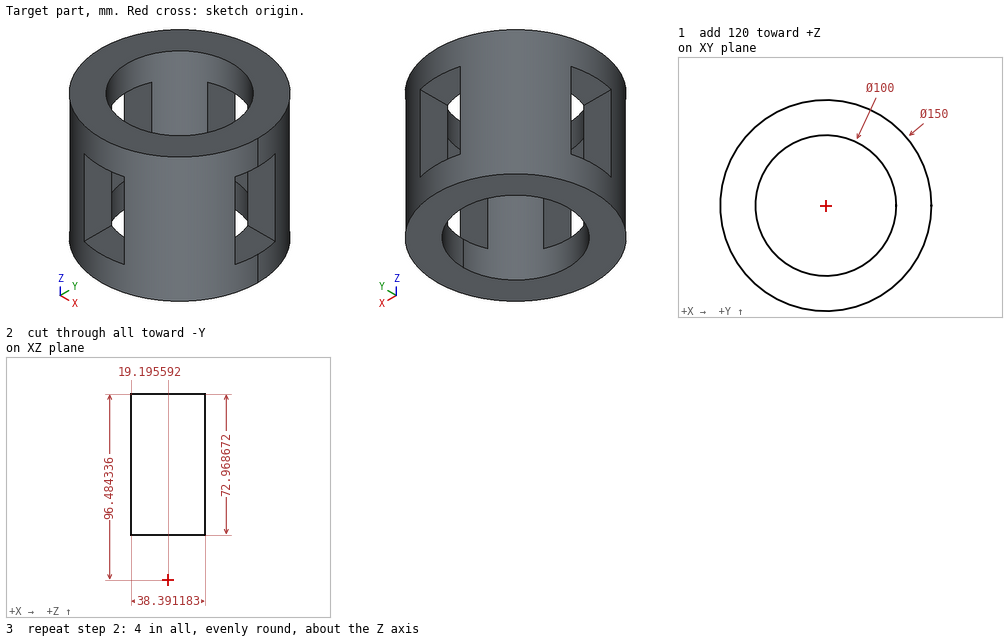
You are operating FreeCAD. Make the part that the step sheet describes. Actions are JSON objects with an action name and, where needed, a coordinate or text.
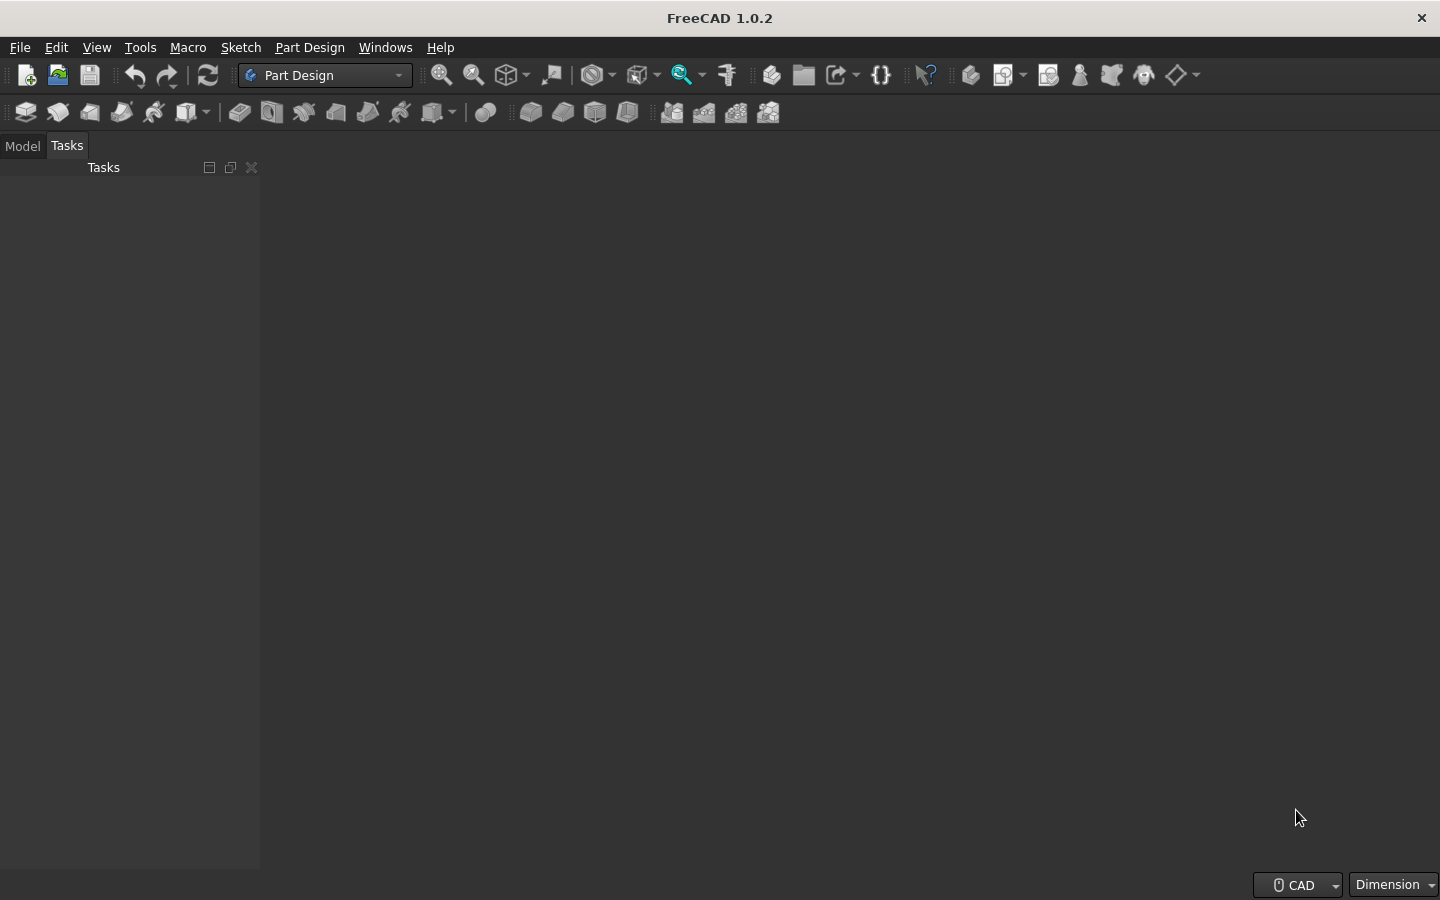
{"action": "left_click", "coordinate": [26, 76]}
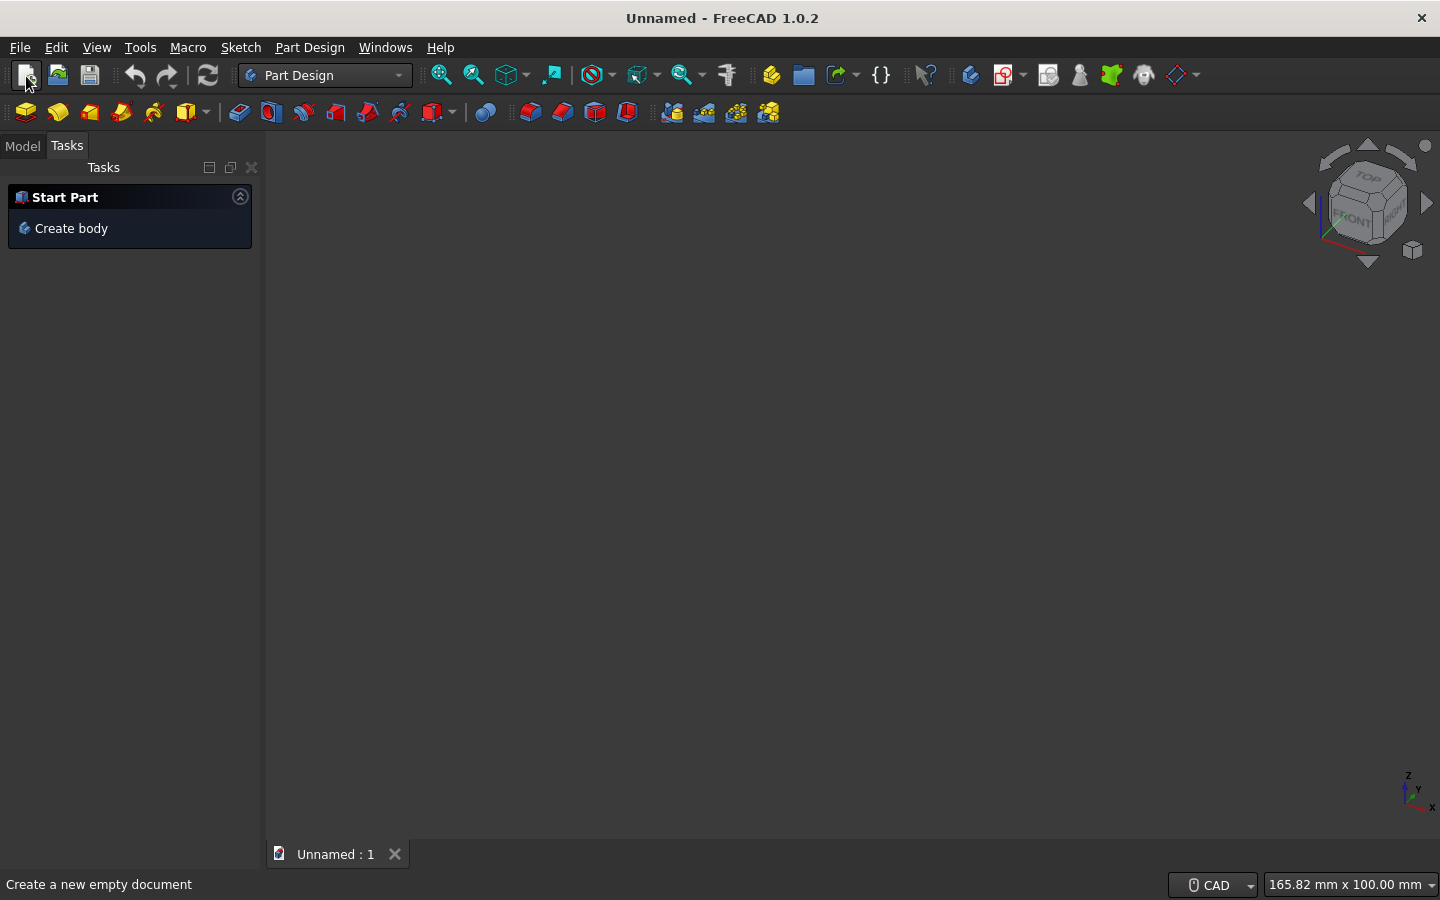
{"action": "left_click", "coordinate": [1004, 76]}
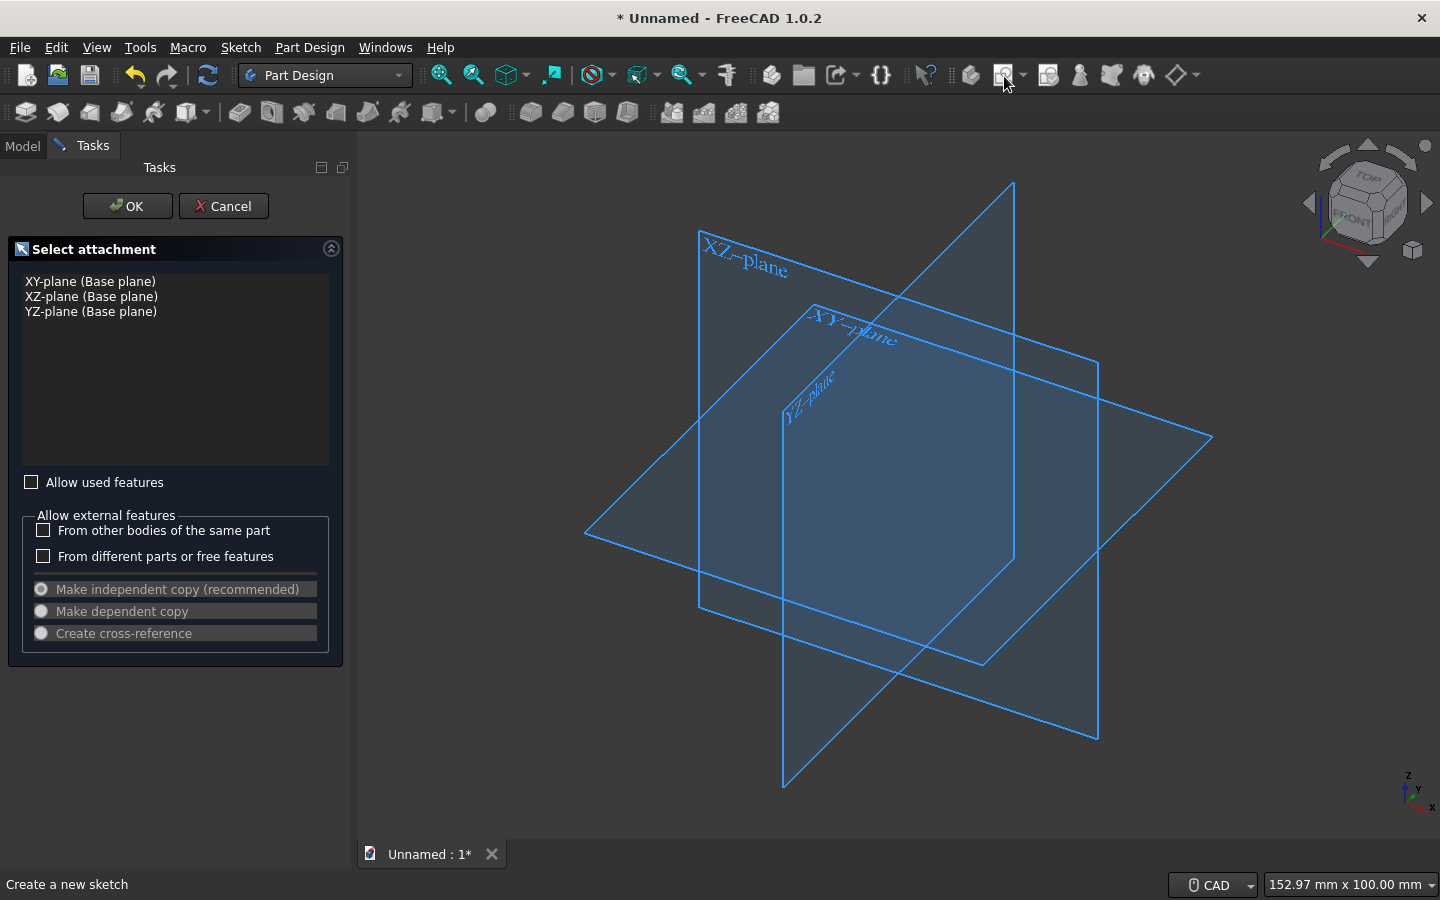
{"action": "left_click", "coordinate": [82, 282]}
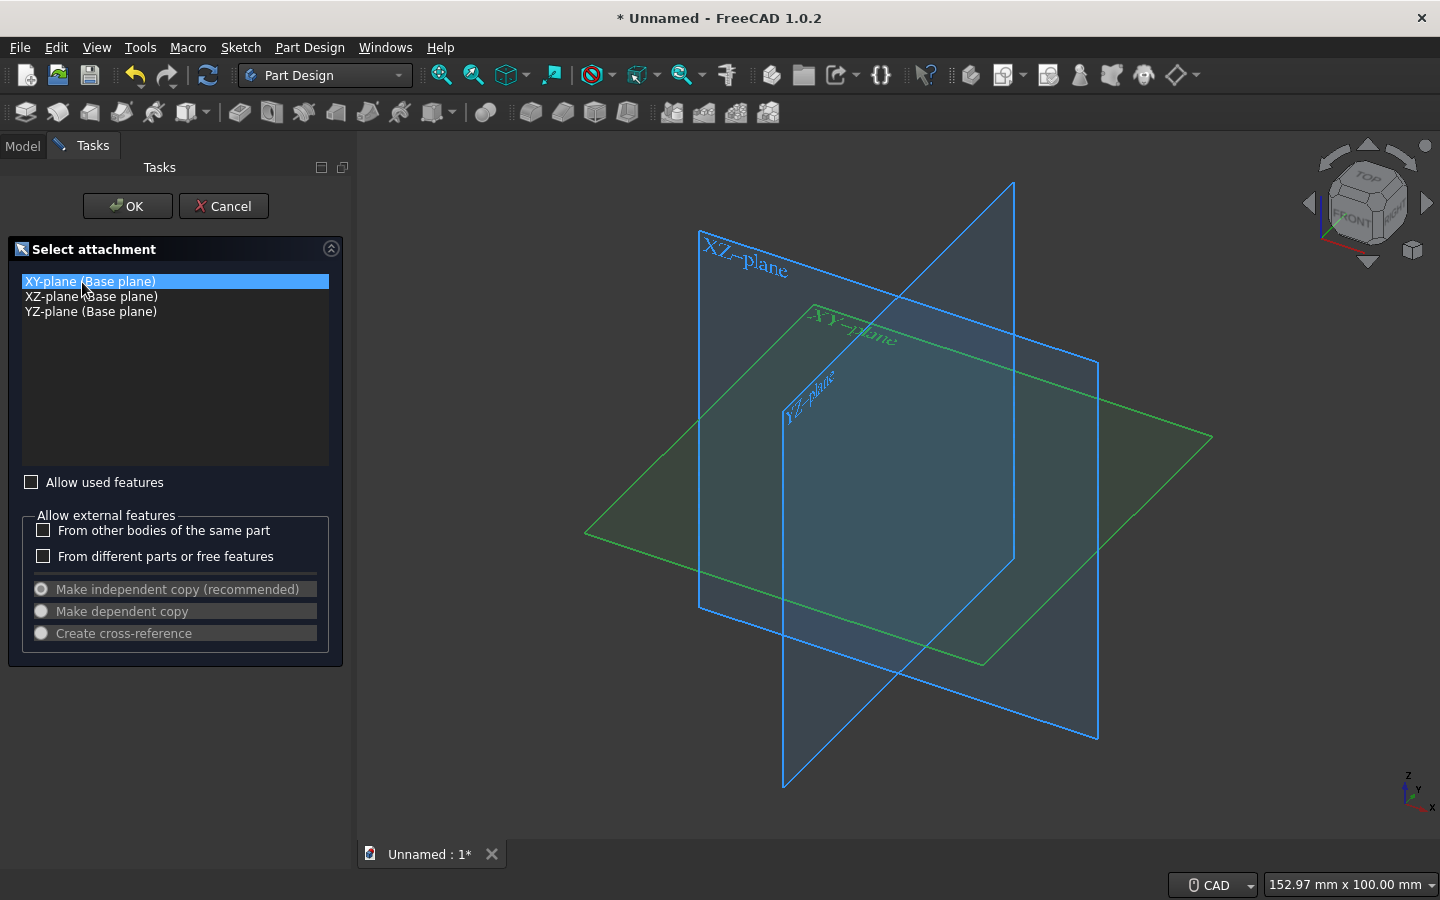
{"action": "left_click", "coordinate": [128, 206]}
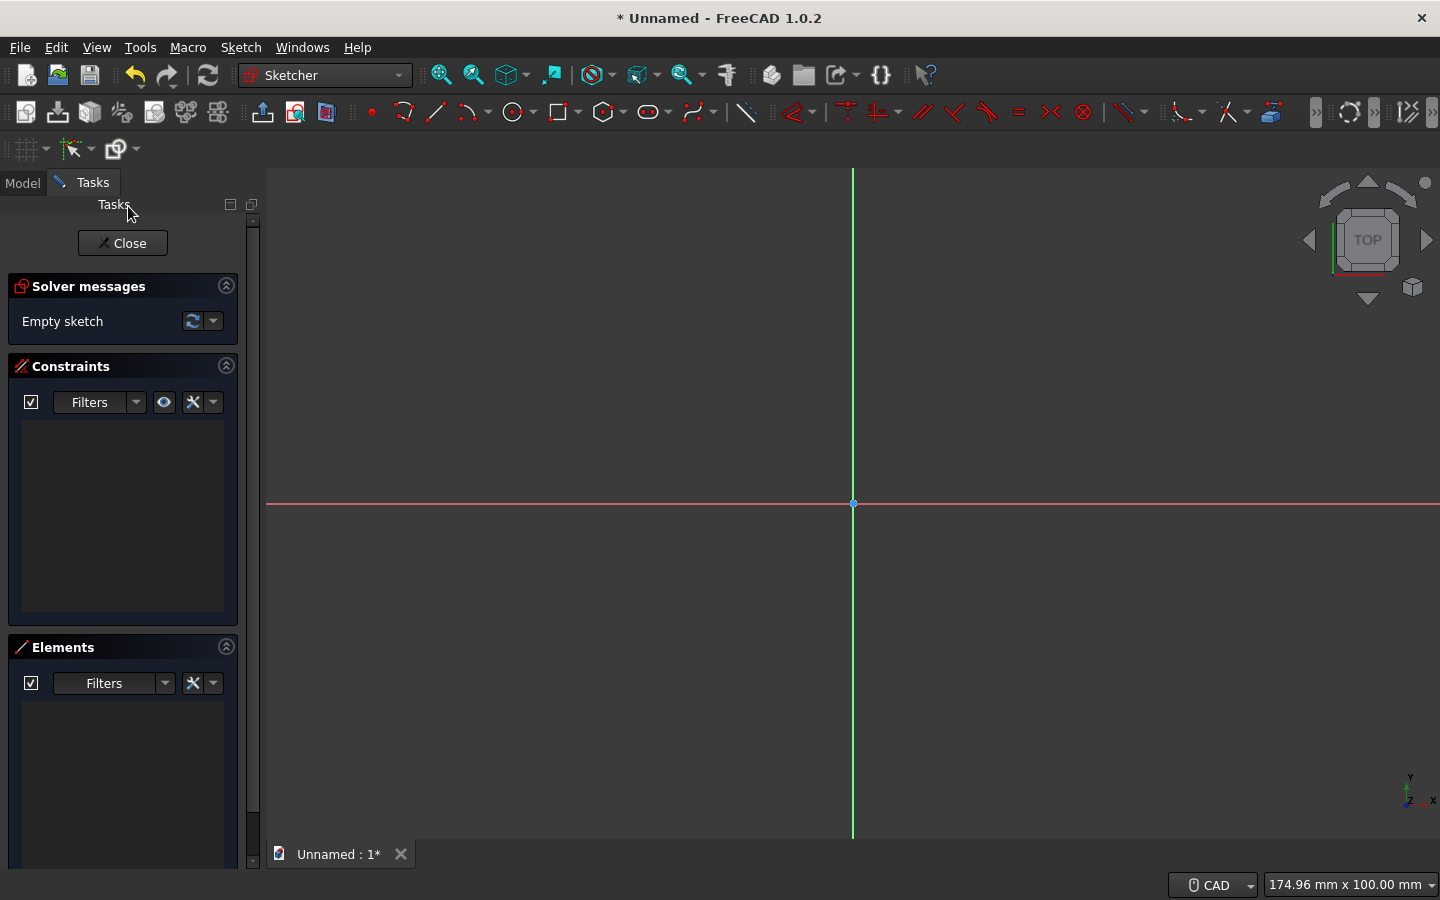
{"action": "scroll", "coordinate": [729, 503], "scroll_direction": "down", "scroll_amount": 4}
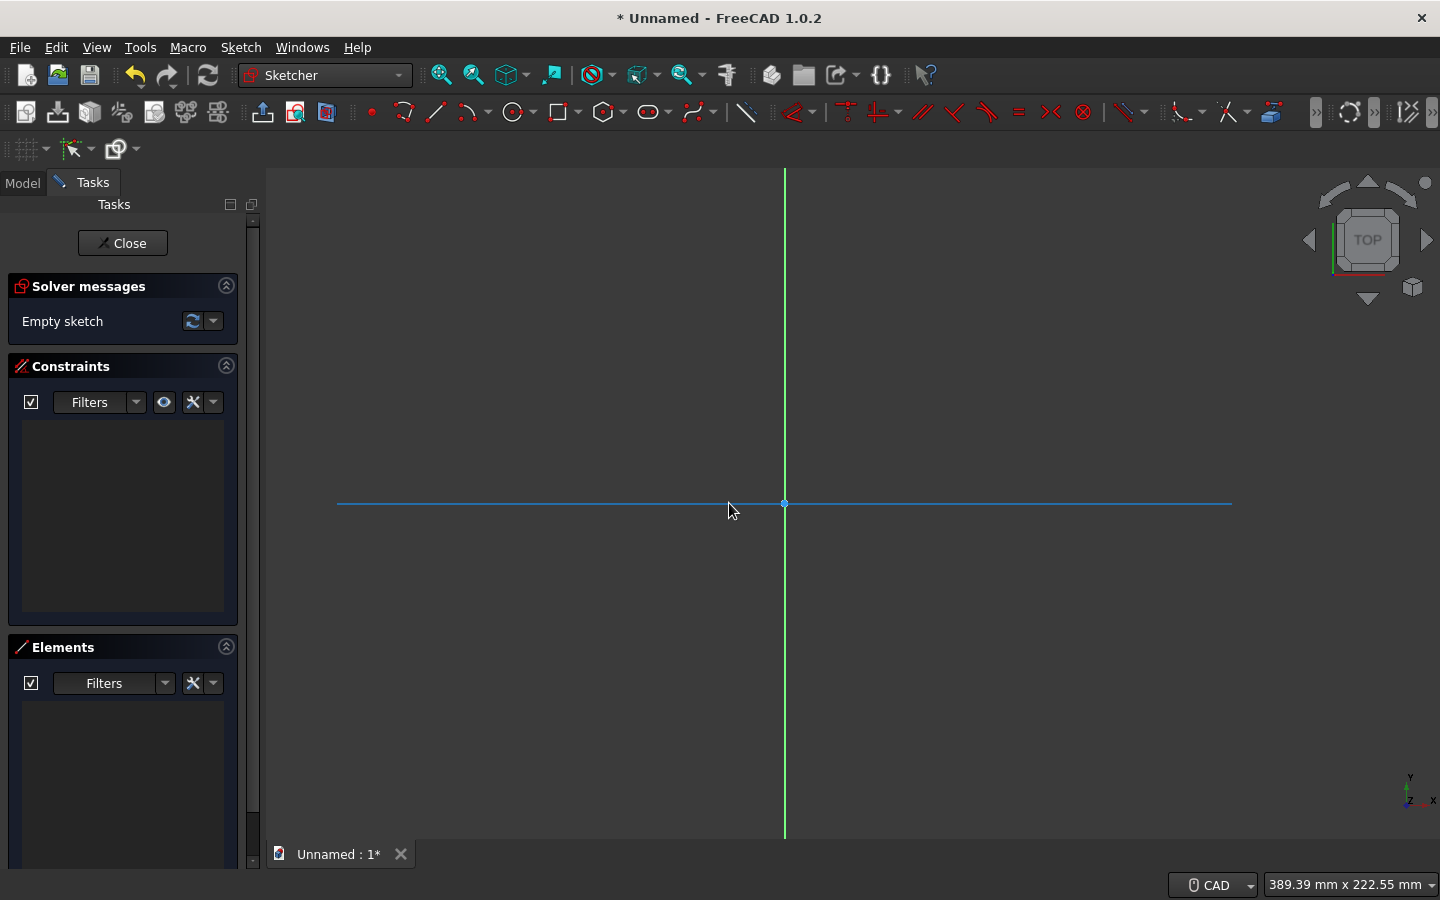
{"action": "left_click", "coordinate": [514, 112]}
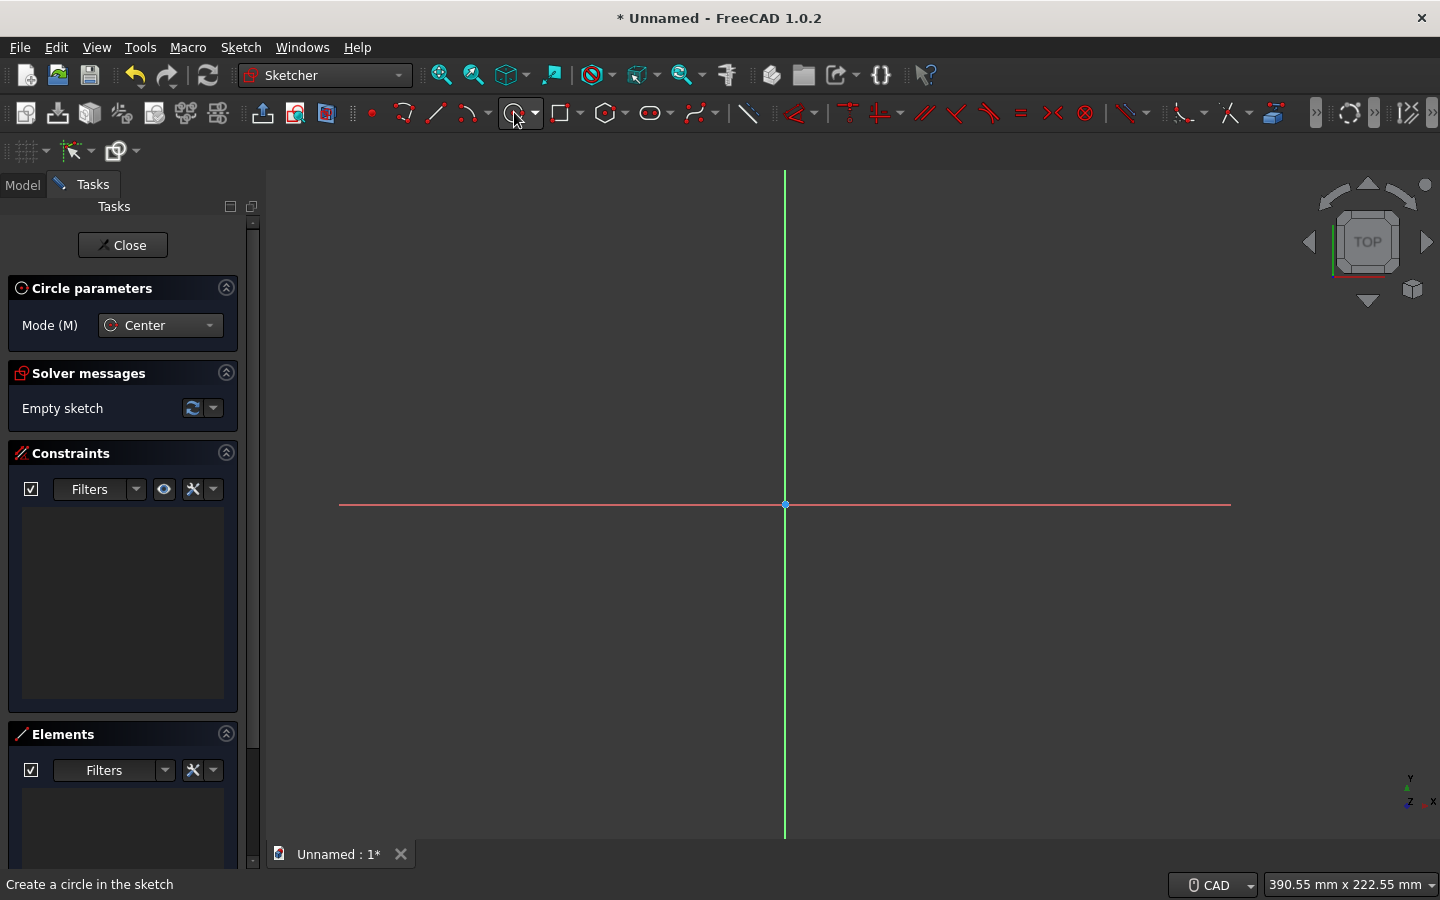
{"action": "left_click", "coordinate": [785, 504]}
{"action": "mouse_move", "coordinate": [945, 345]}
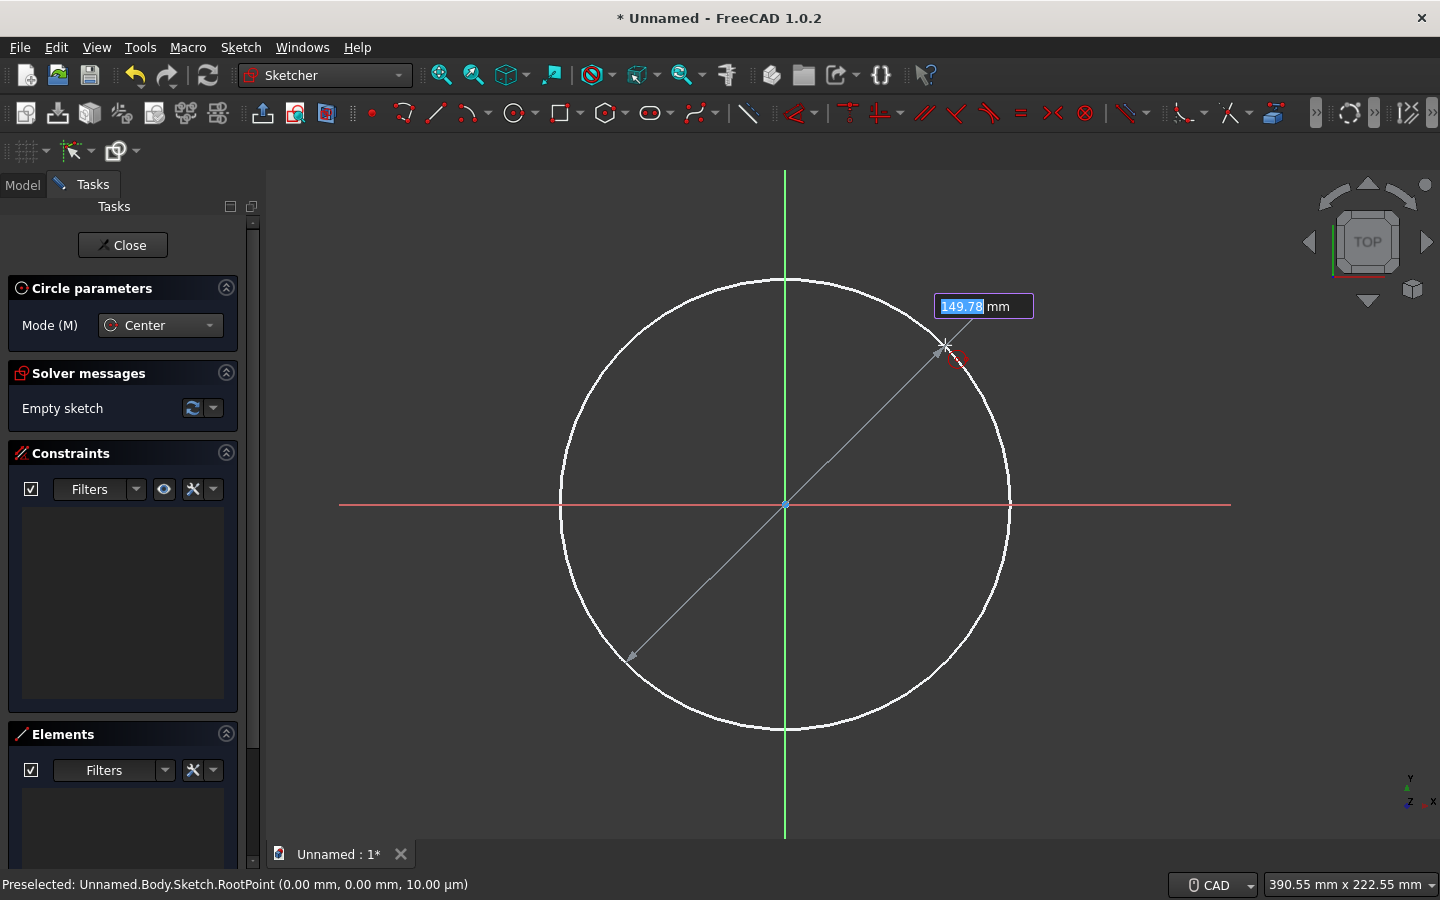
{"action": "type", "text": "150"}
{"action": "key", "text": "Return"}